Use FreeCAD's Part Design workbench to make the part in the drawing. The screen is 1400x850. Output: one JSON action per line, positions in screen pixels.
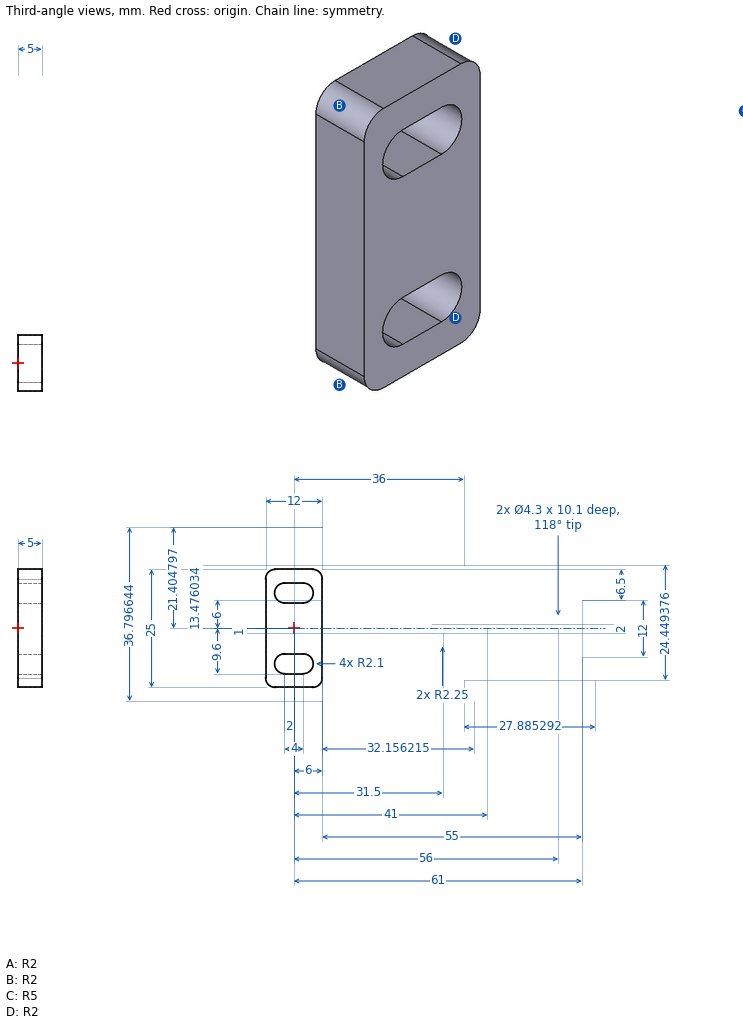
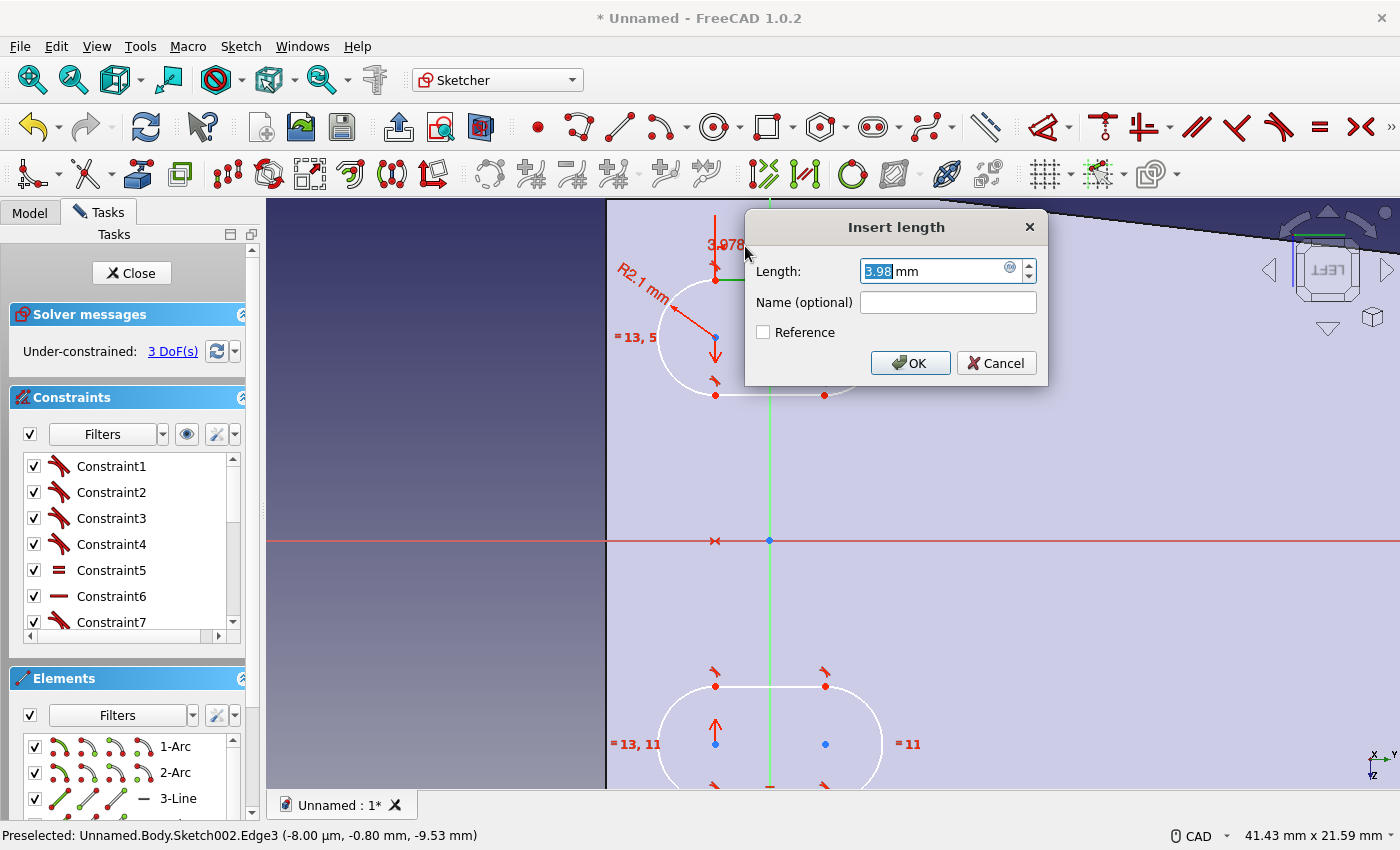
{"action": "type", "text": "4"}
{"action": "key", "text": "Return"}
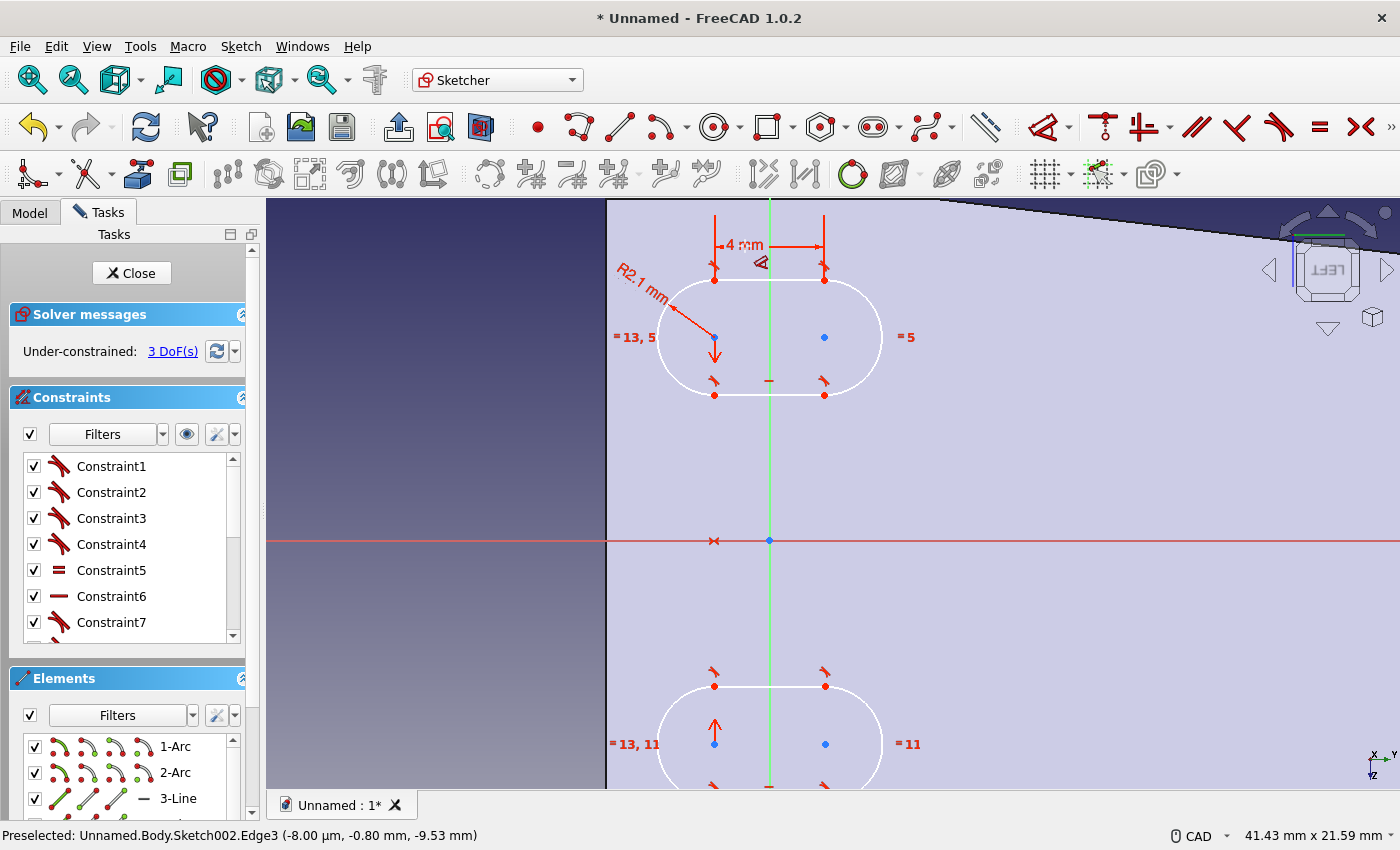
{"action": "left_click", "coordinate": [748, 687]}
{"action": "left_click", "coordinate": [745, 721]}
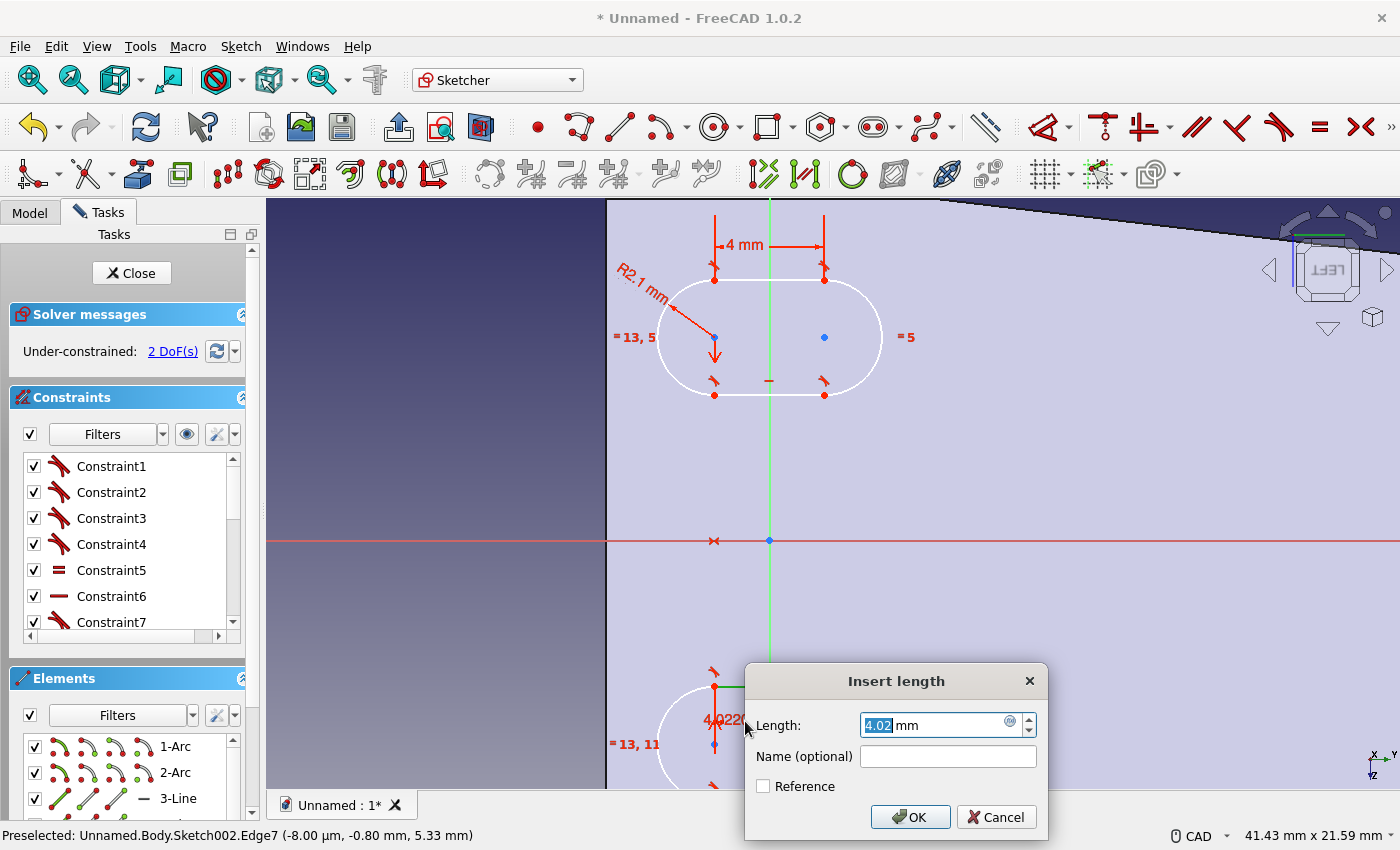
{"action": "type", "text": "4"}
{"action": "key", "text": "Return"}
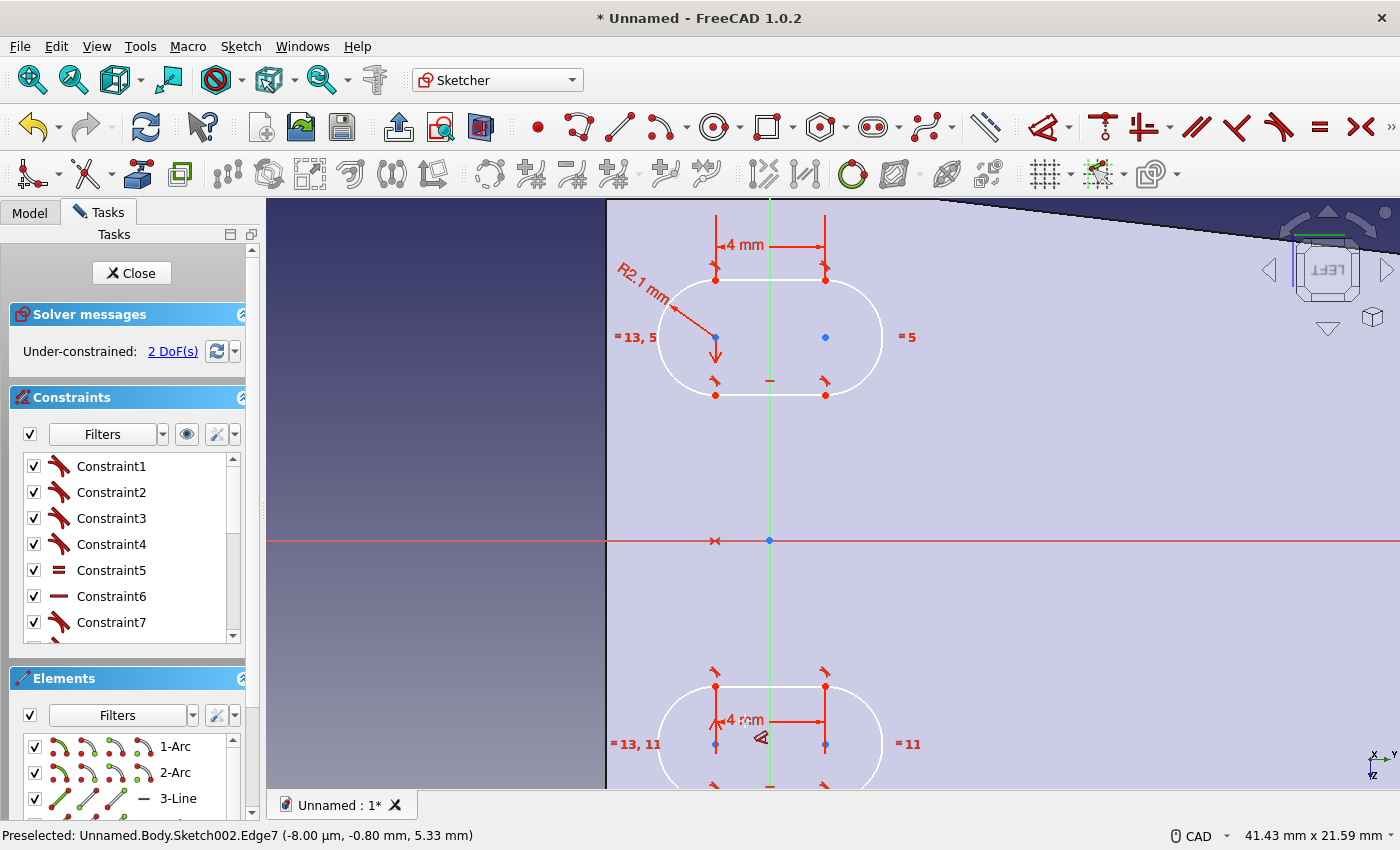
{"action": "left_click", "coordinate": [716, 280]}
{"action": "left_click", "coordinate": [743, 575]}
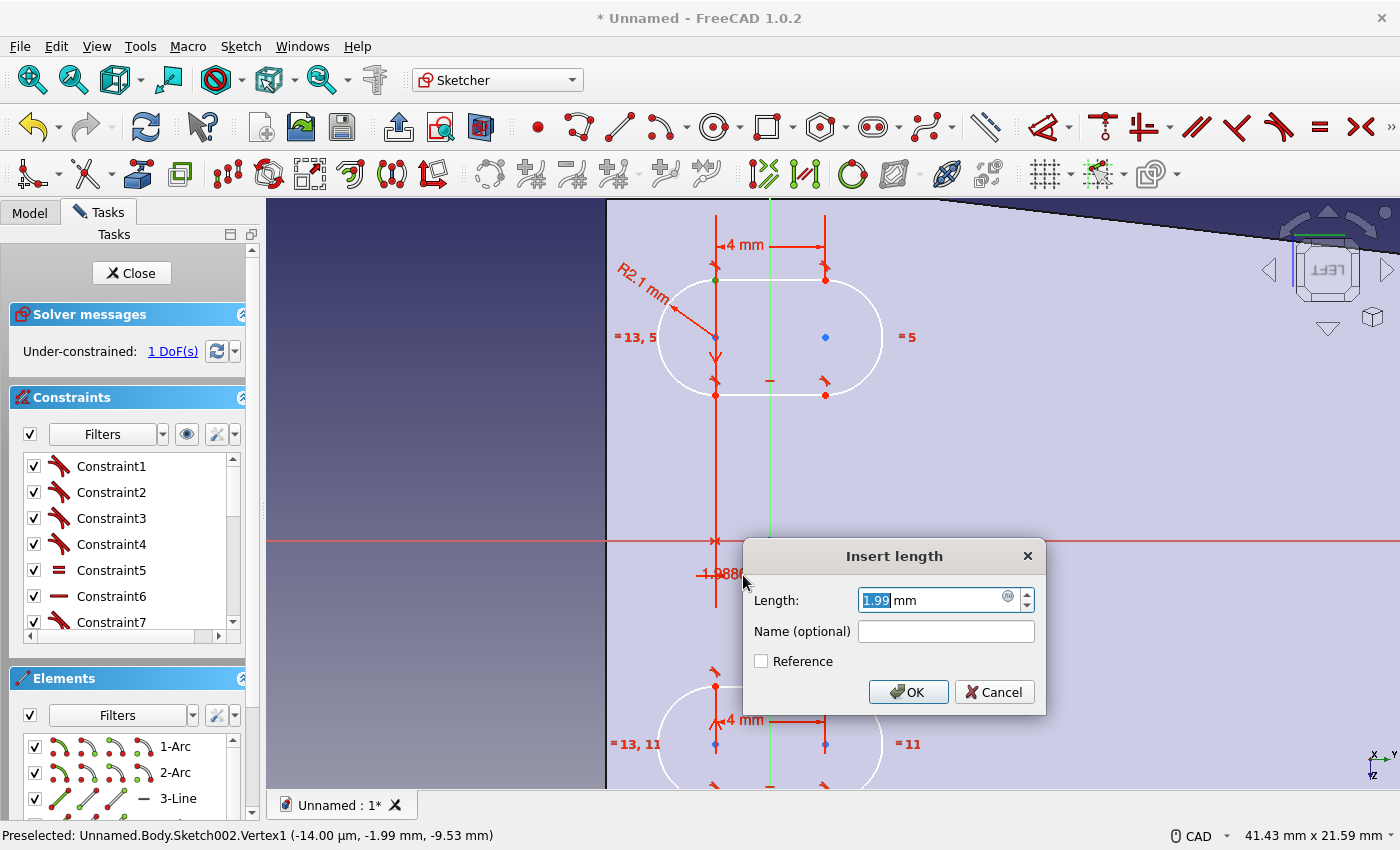
{"action": "type", "text": "2"}
{"action": "key", "text": "Return"}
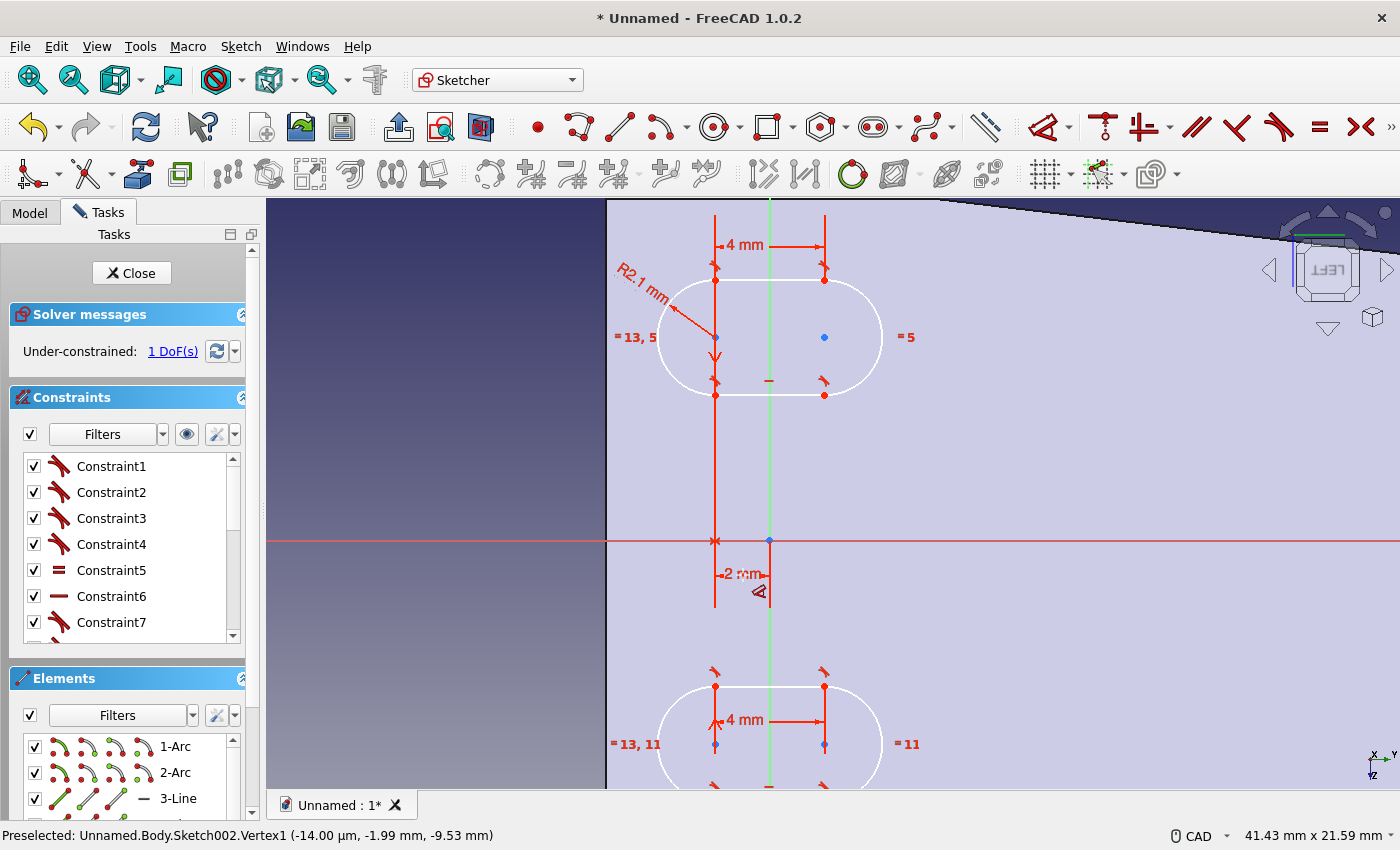
{"action": "left_click", "coordinate": [715, 280]}
{"action": "left_click", "coordinate": [681, 411]}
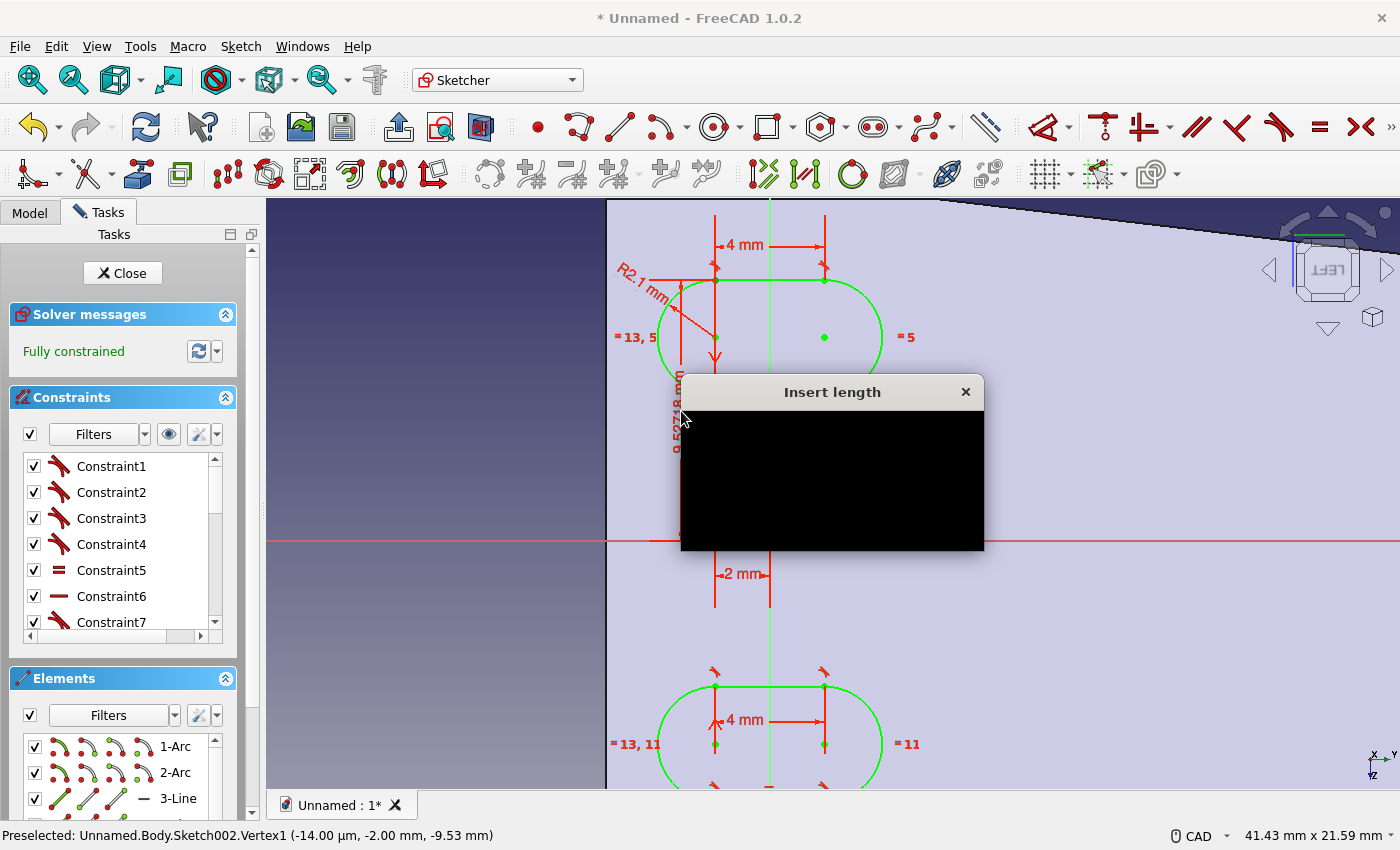
{"action": "type", "text": "9.6"}
{"action": "key", "text": "Return"}
{"action": "key", "text": "Escape"}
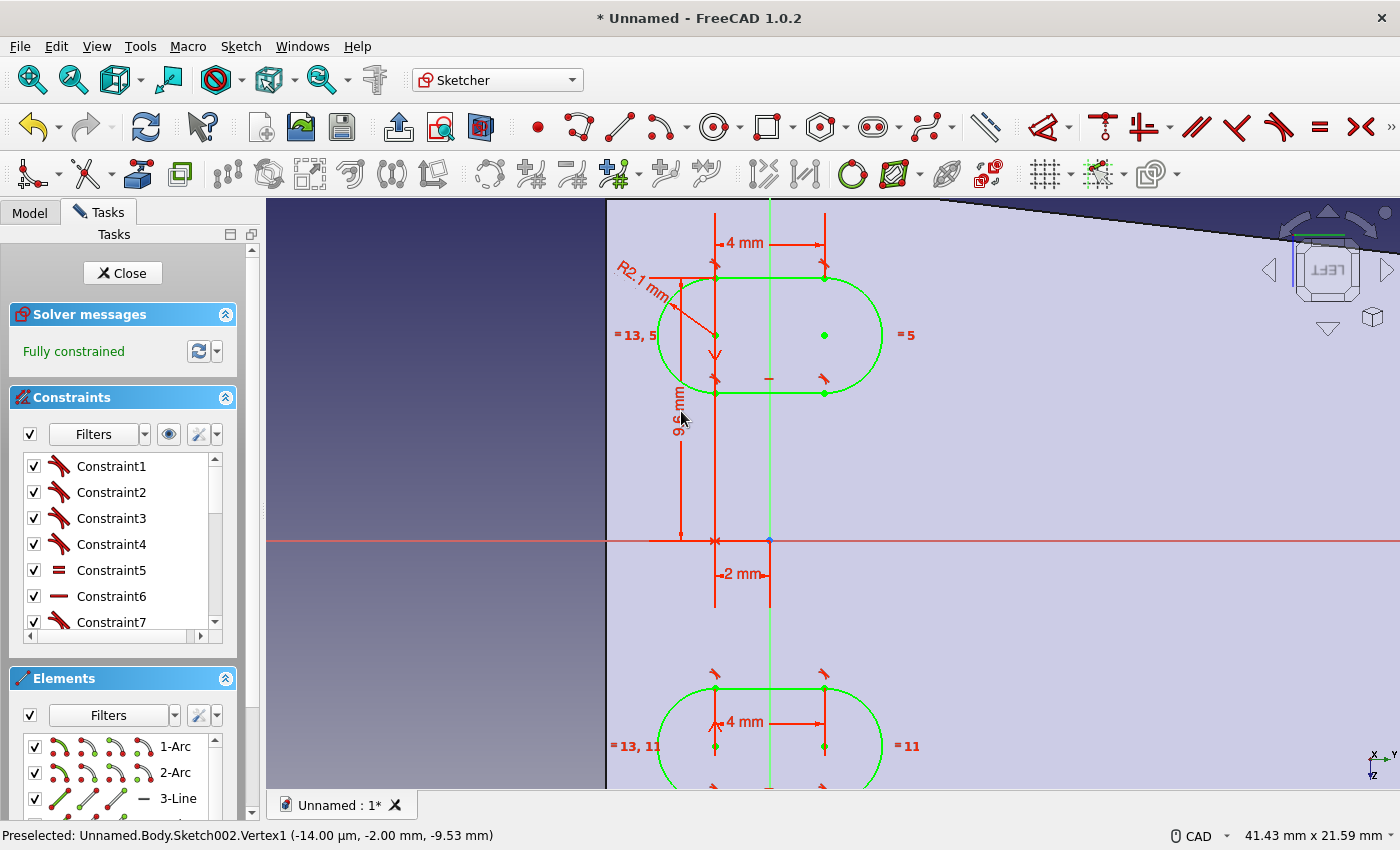
{"action": "left_click", "coordinate": [123, 273]}